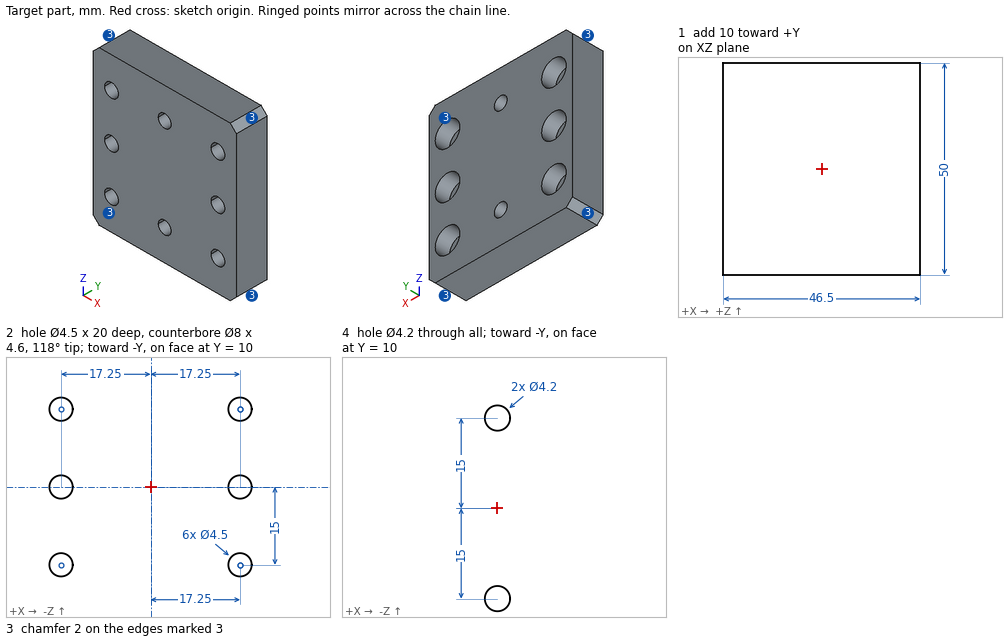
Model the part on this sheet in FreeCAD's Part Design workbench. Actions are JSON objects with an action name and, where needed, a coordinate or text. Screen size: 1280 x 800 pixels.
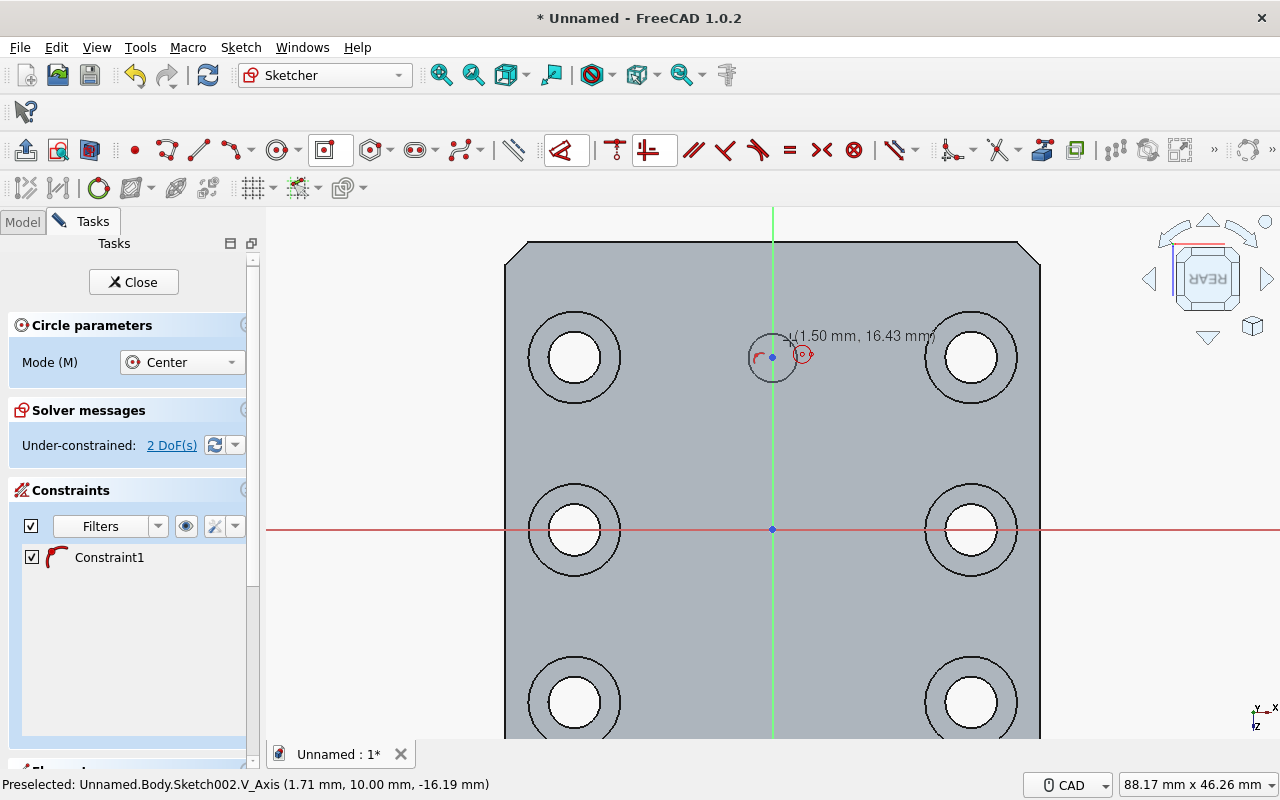
{"action": "left_click", "coordinate": [773, 702]}
{"action": "left_click", "coordinate": [790, 685]}
{"action": "key", "text": "Escape"}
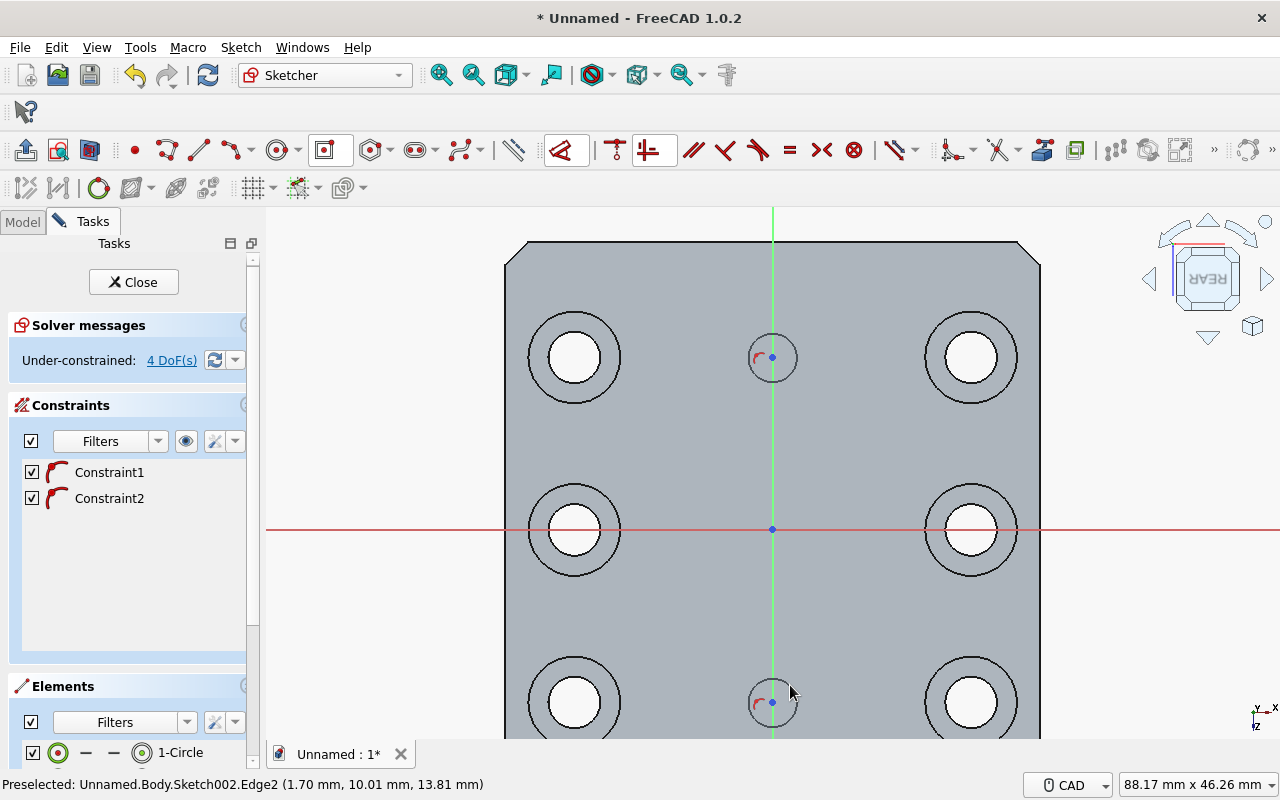
{"action": "left_click", "coordinate": [790, 341]}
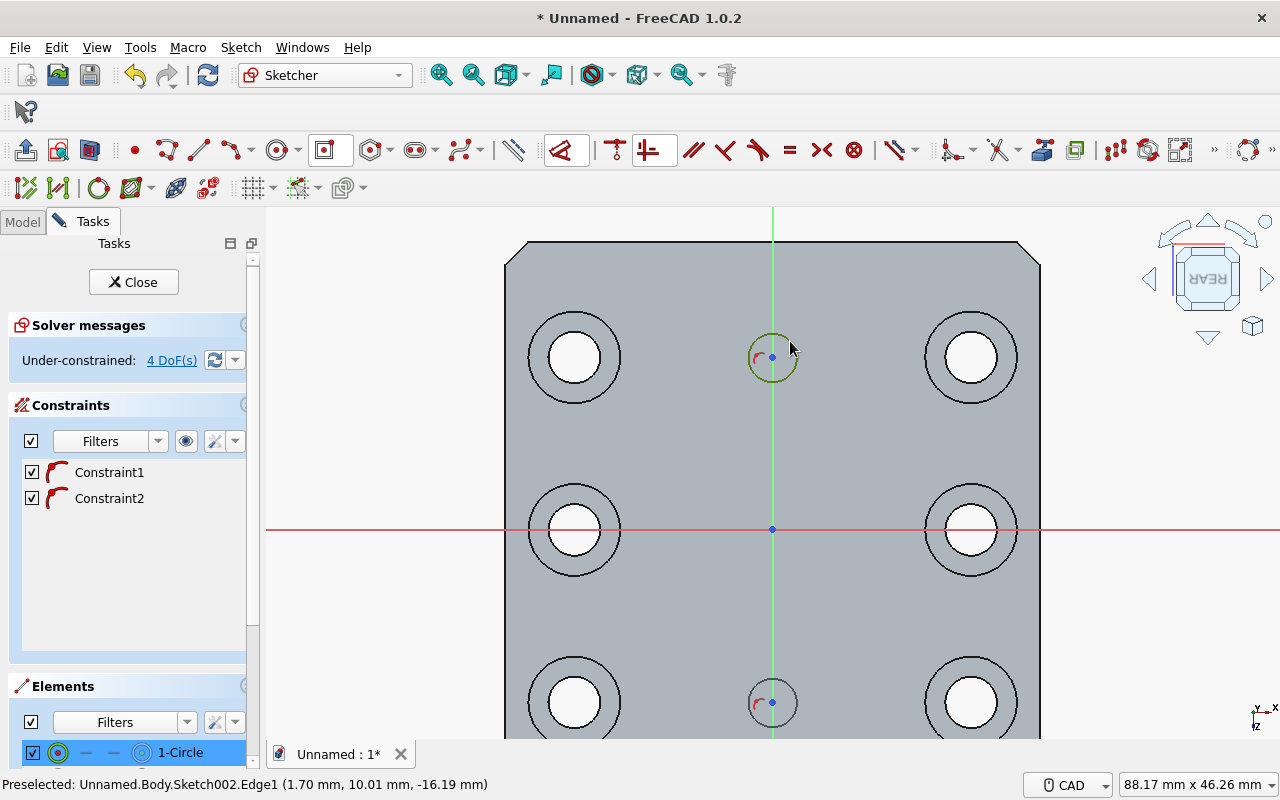
{"action": "left_click", "coordinate": [790, 686]}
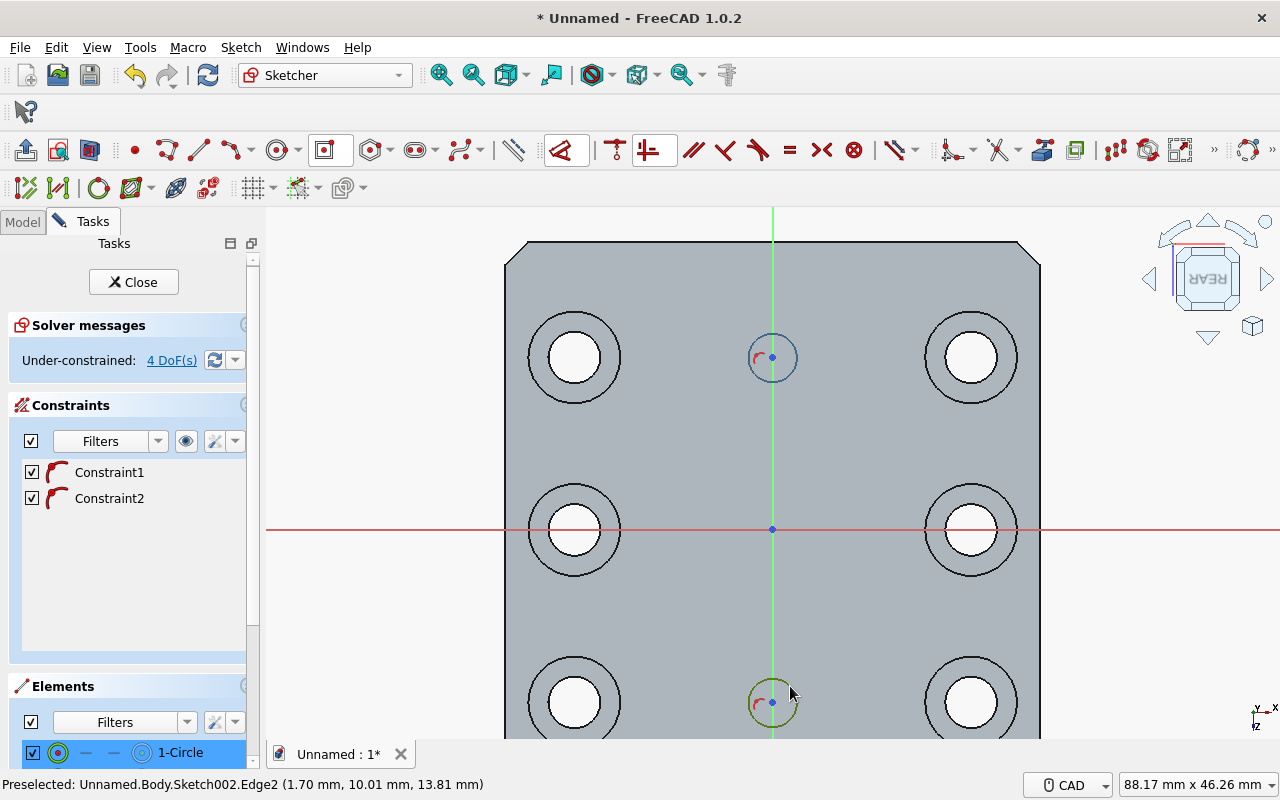
{"action": "left_click", "coordinate": [790, 150]}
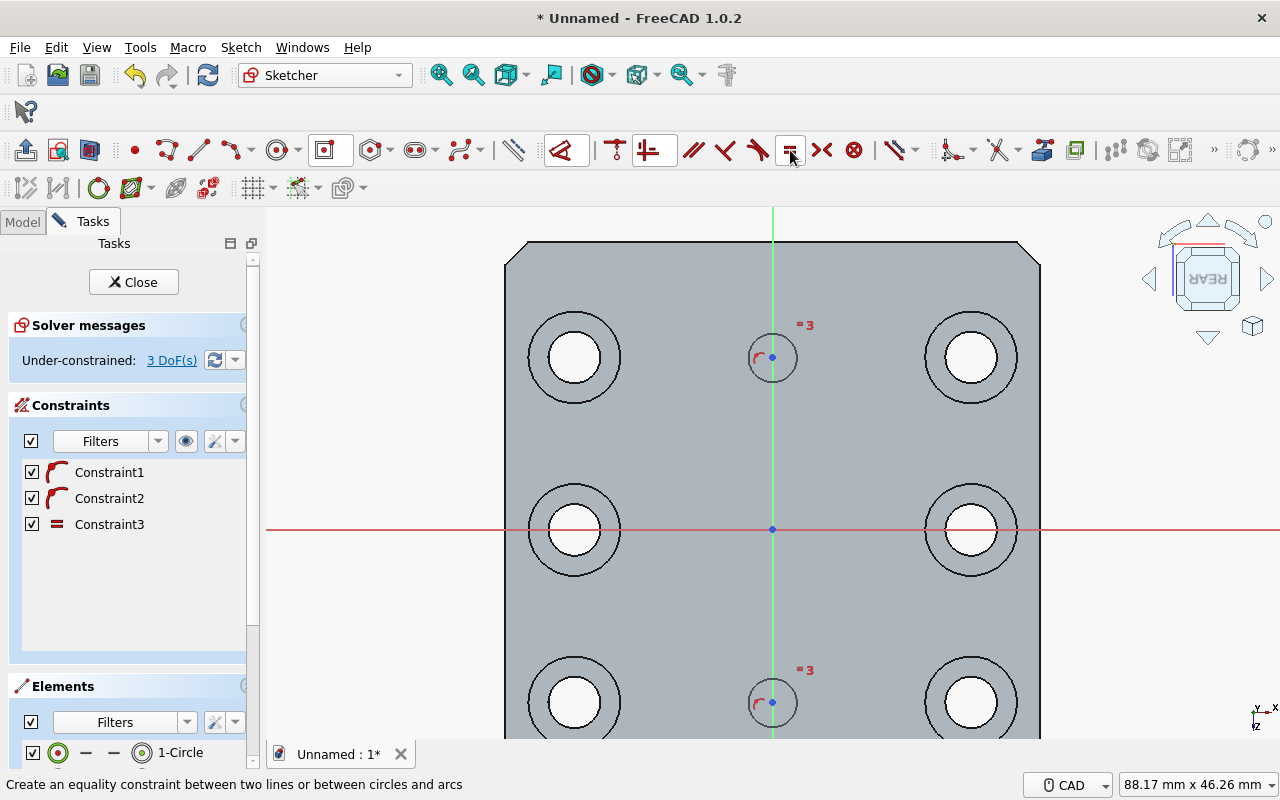
{"action": "left_click", "coordinate": [790, 341]}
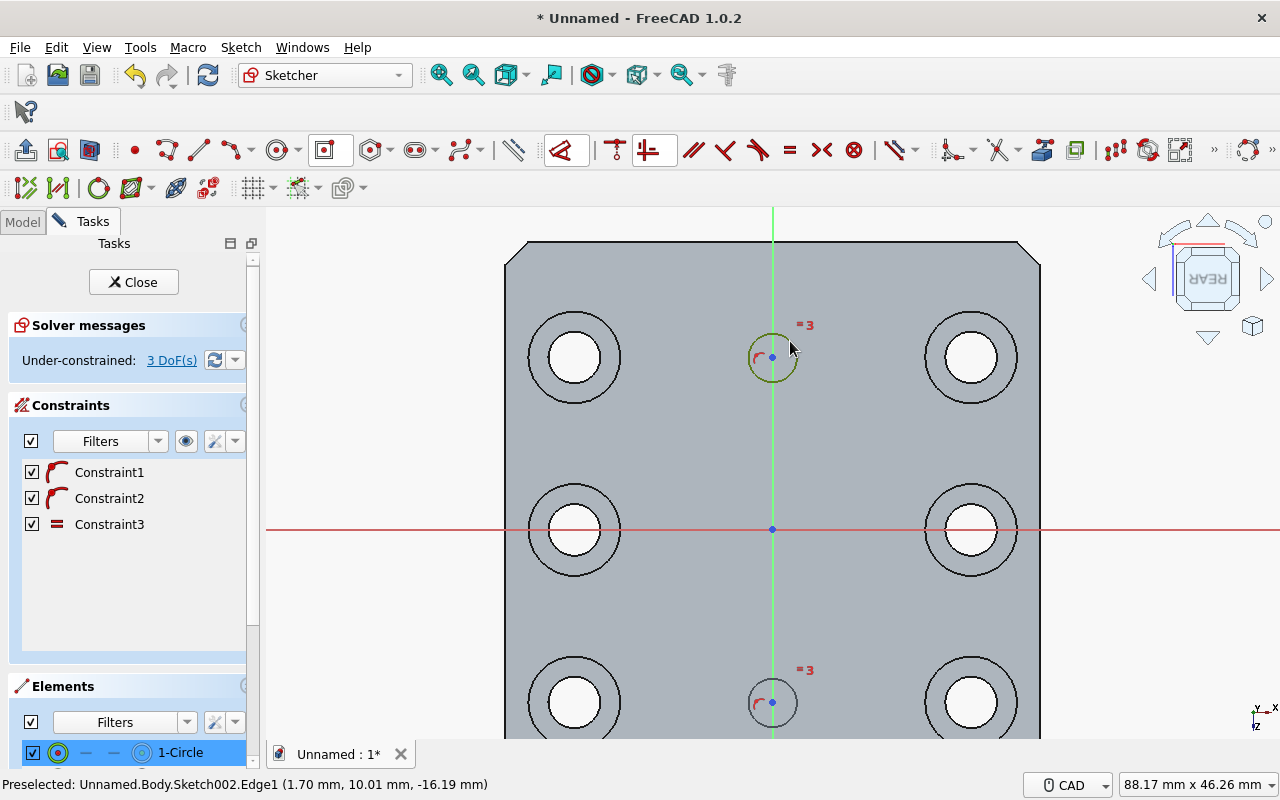
{"action": "key", "text": "k o"}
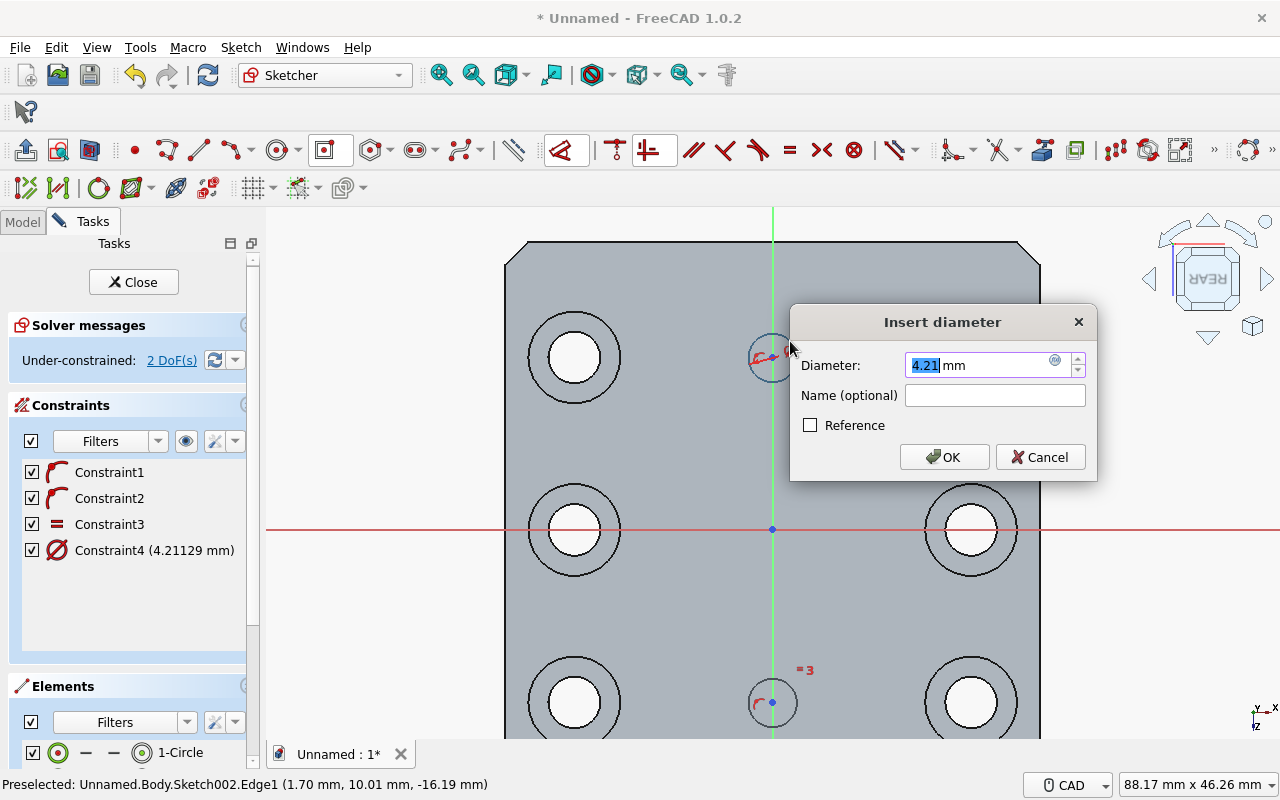
{"action": "type", "text": "4.2"}
{"action": "key", "text": "Return"}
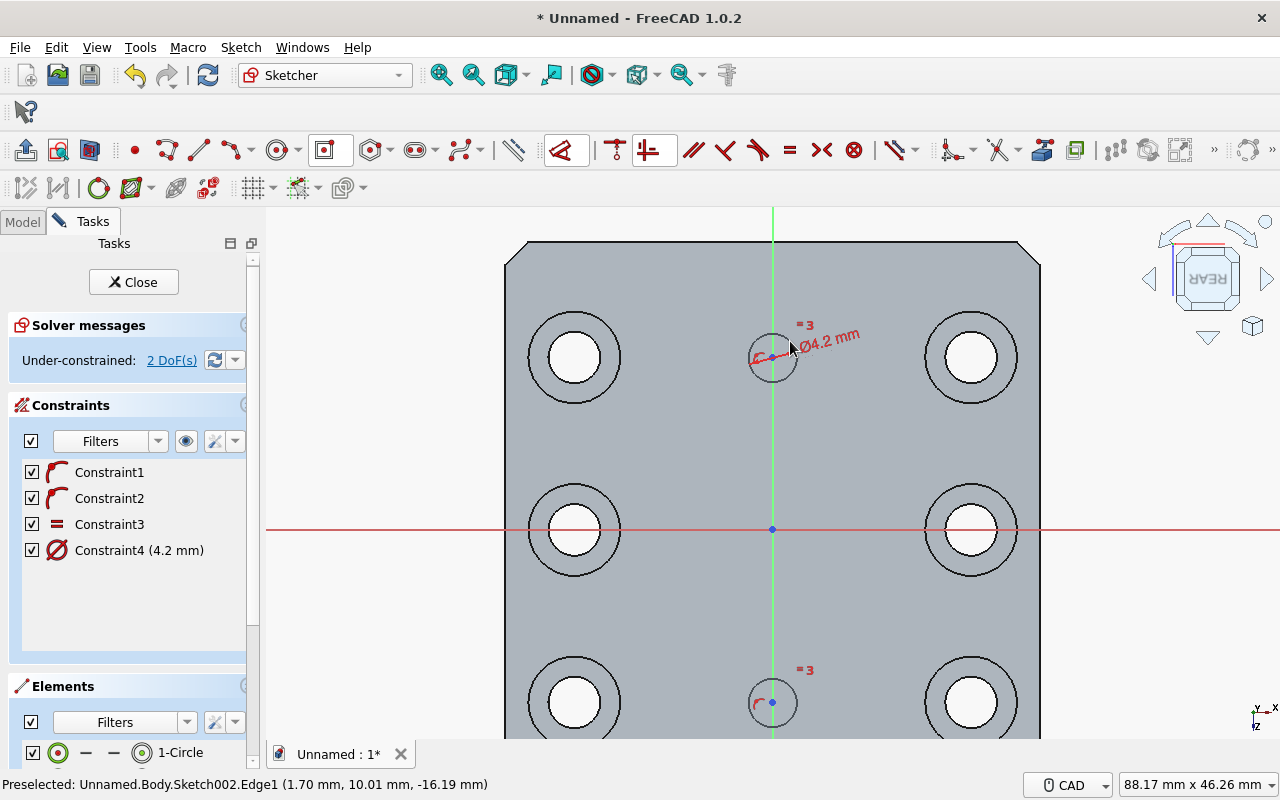
{"action": "left_click", "coordinate": [773, 358]}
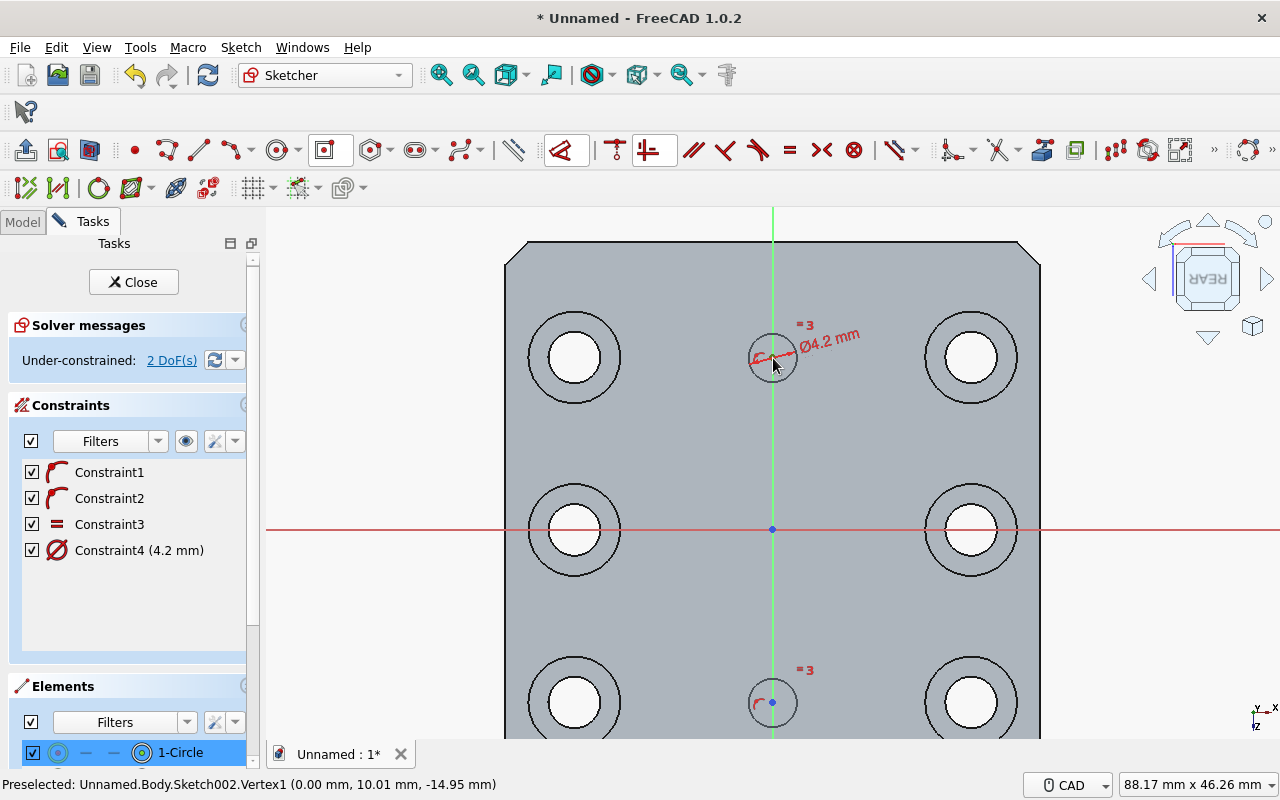
{"action": "key", "text": "i"}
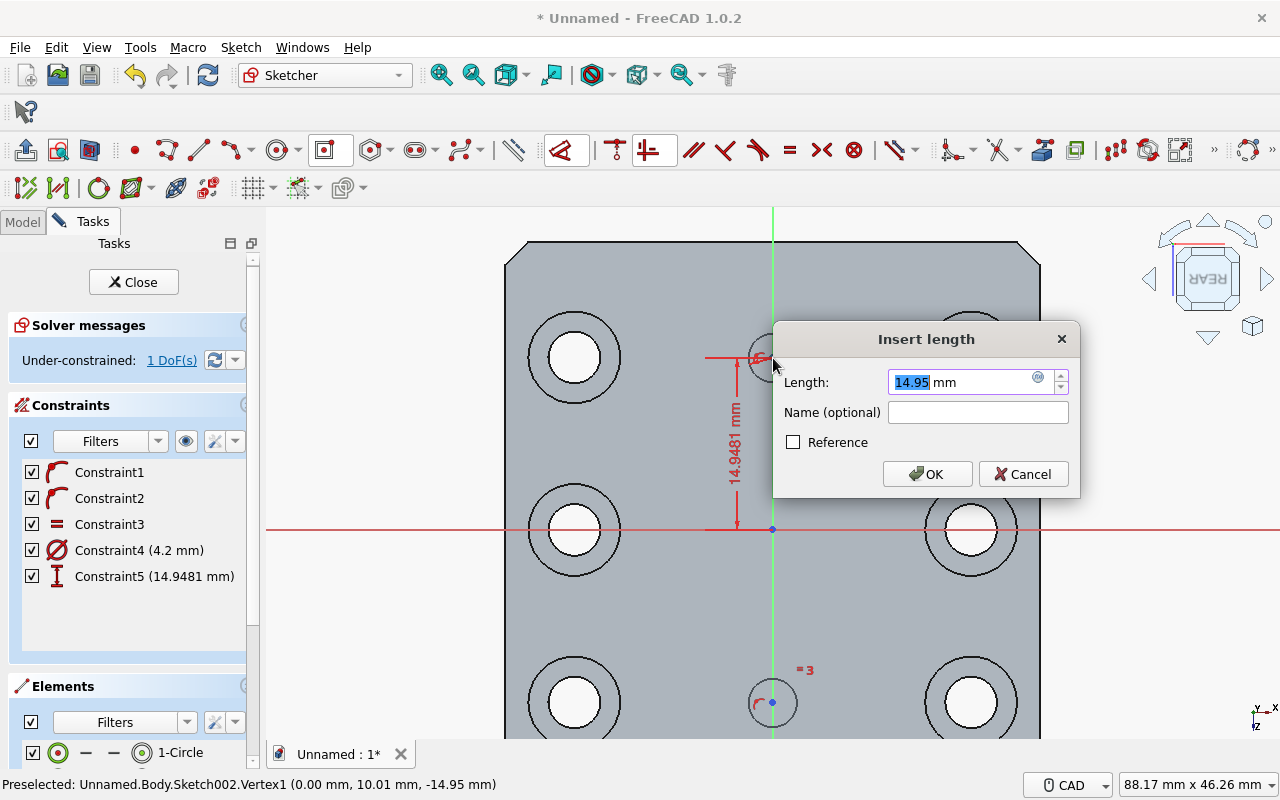
{"action": "type", "text": "15"}
{"action": "key", "text": "Return"}